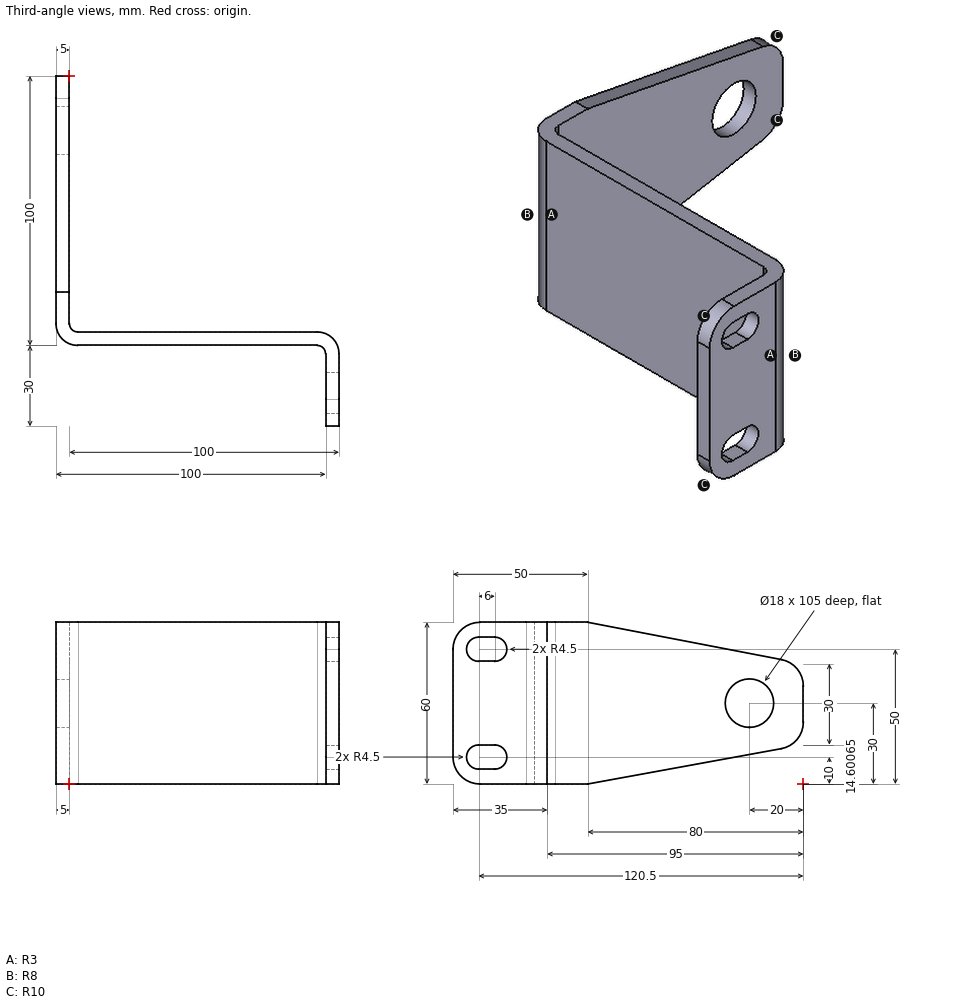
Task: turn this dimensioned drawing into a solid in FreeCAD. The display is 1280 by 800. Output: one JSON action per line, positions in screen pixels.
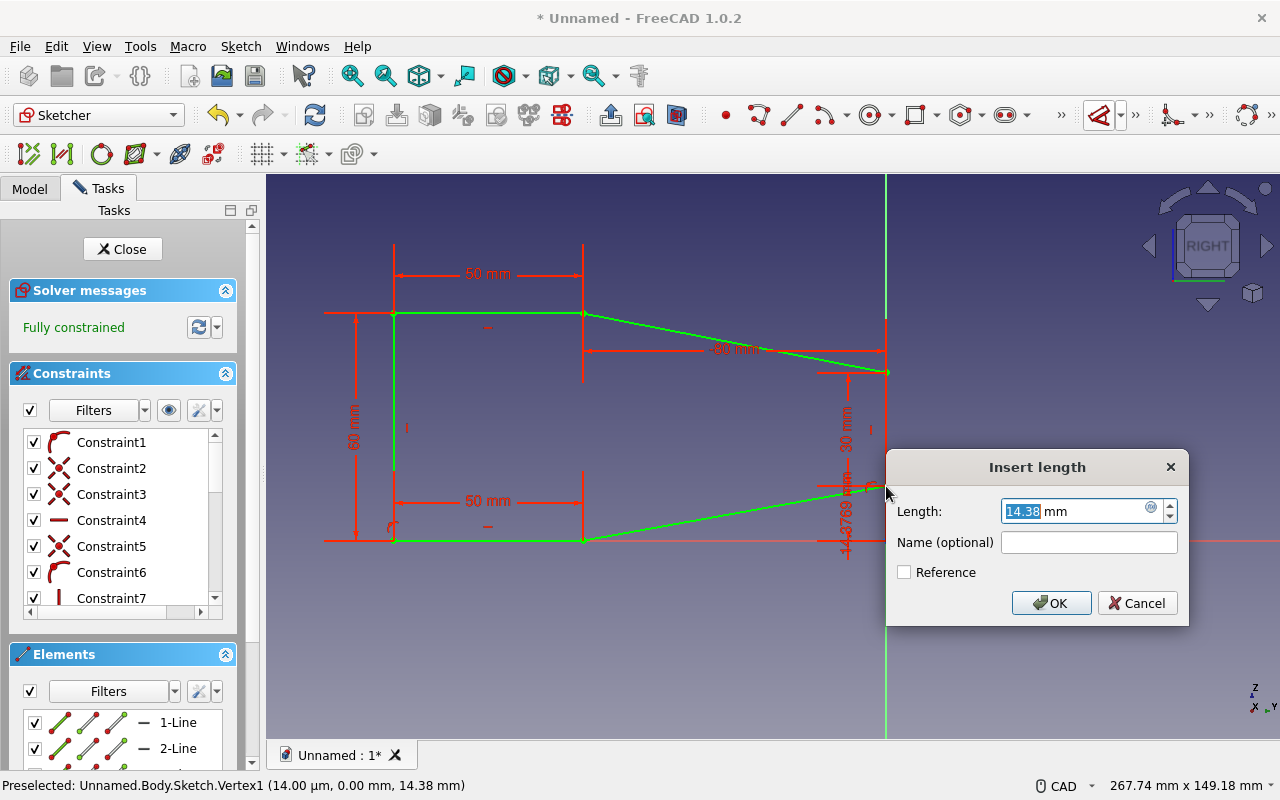
{"action": "type", "text": "14.60065"}
{"action": "key", "text": "Return"}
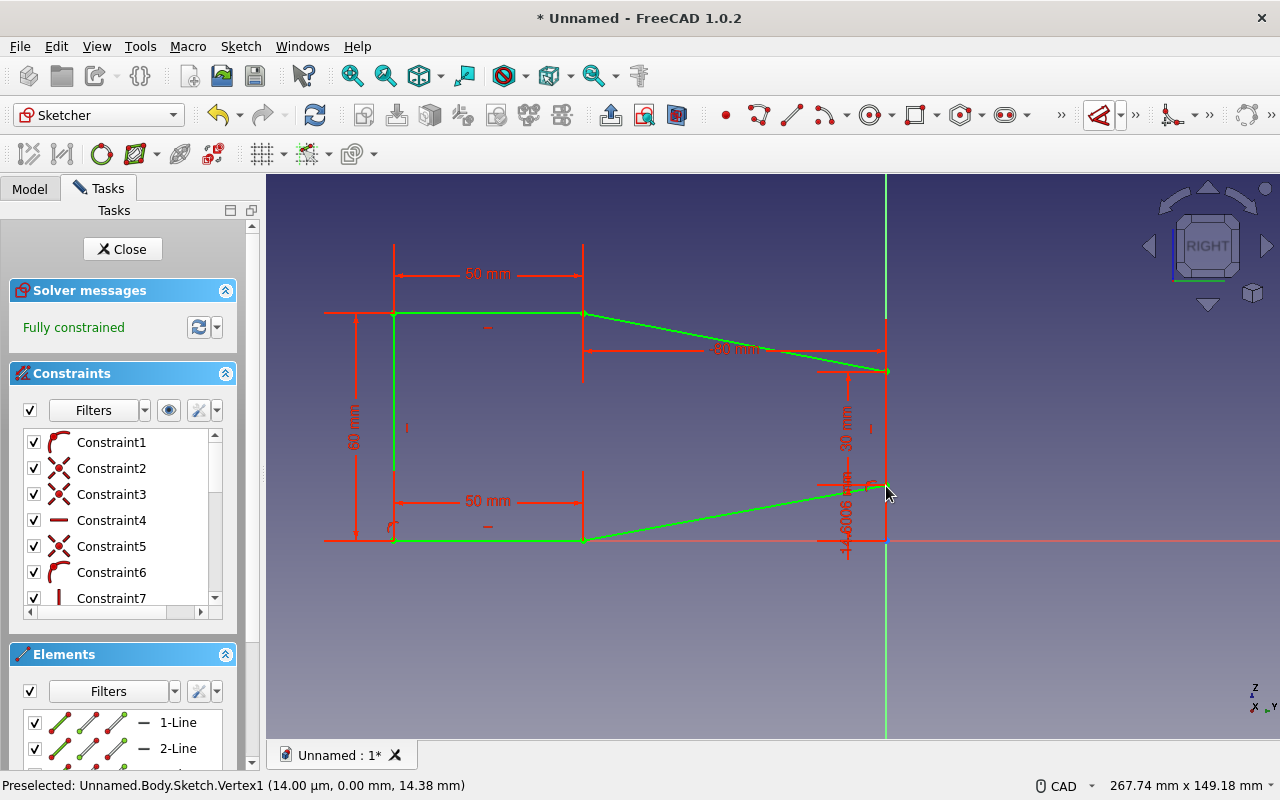
{"action": "left_click", "coordinate": [123, 249]}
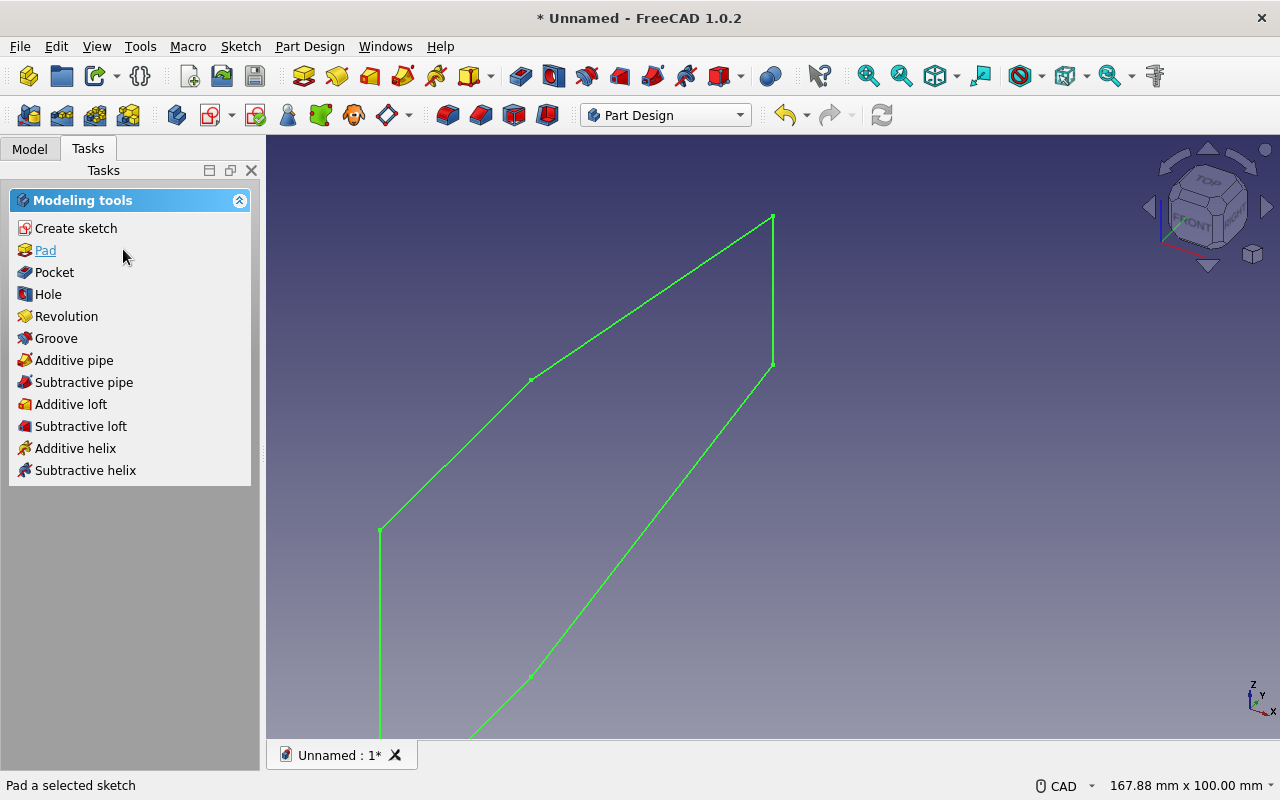
{"action": "left_click", "coordinate": [304, 76]}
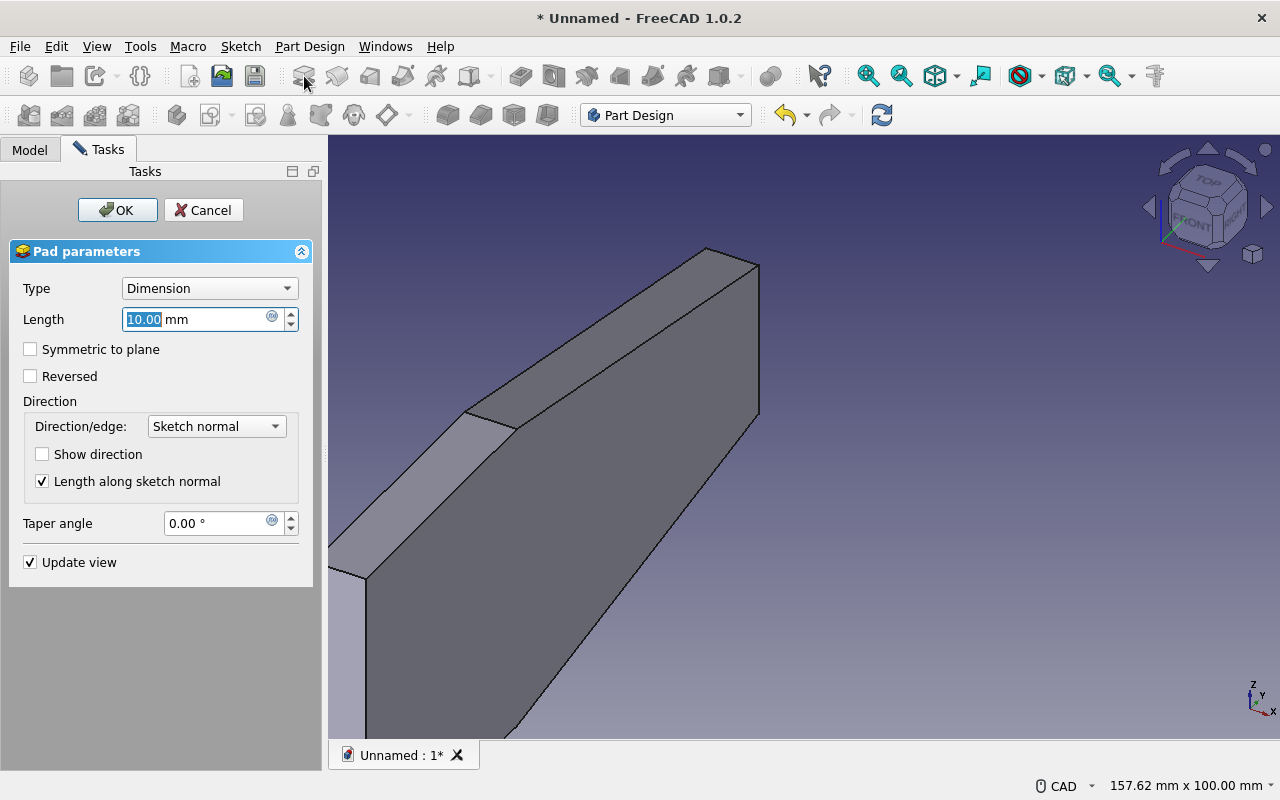
{"action": "type", "text": "5"}
{"action": "key", "text": "Tab"}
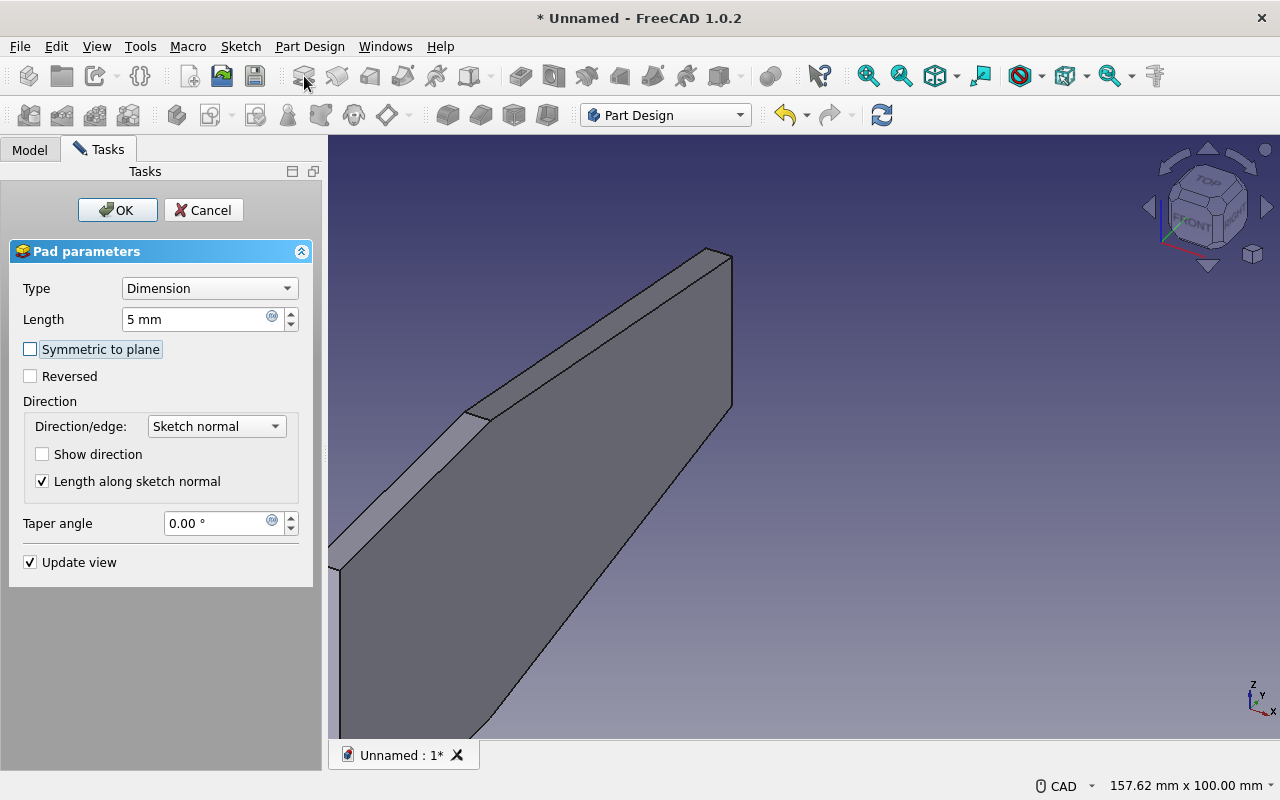
{"action": "left_click", "coordinate": [31, 376]}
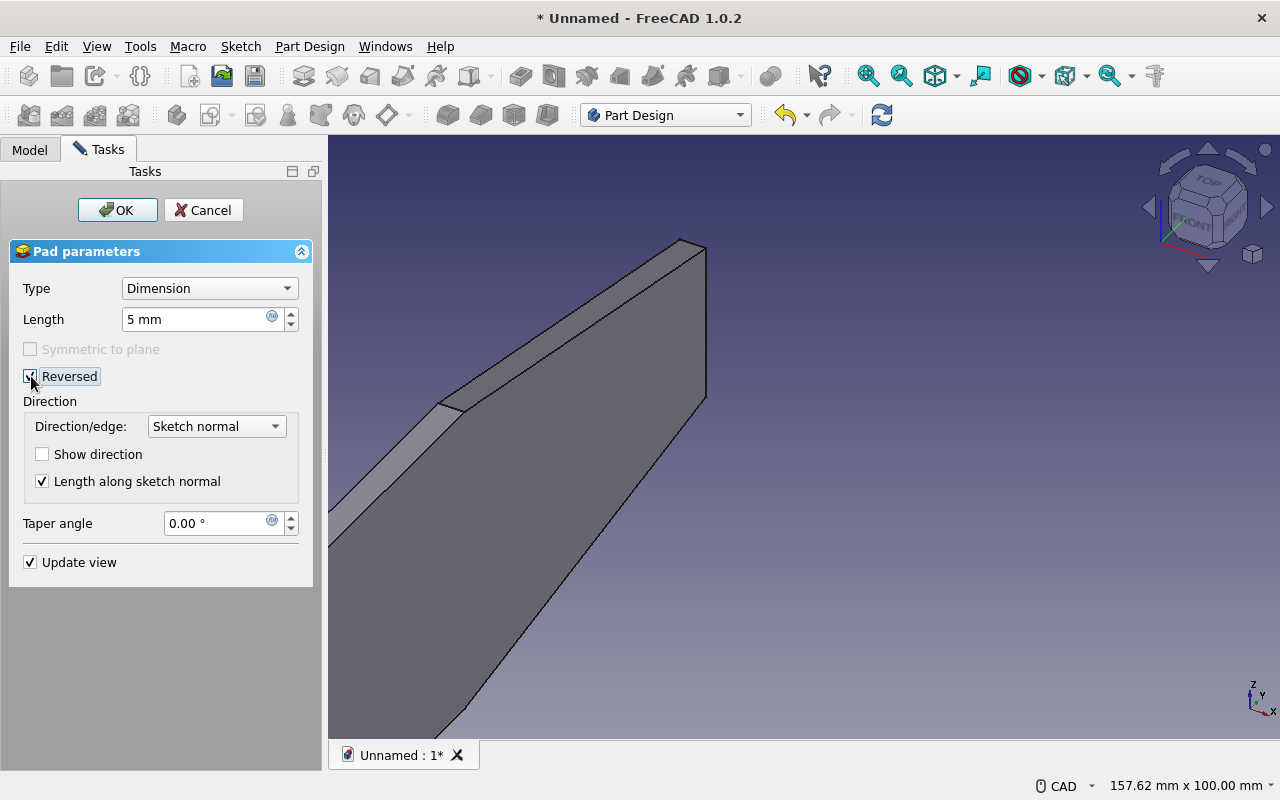
{"action": "left_click", "coordinate": [118, 210]}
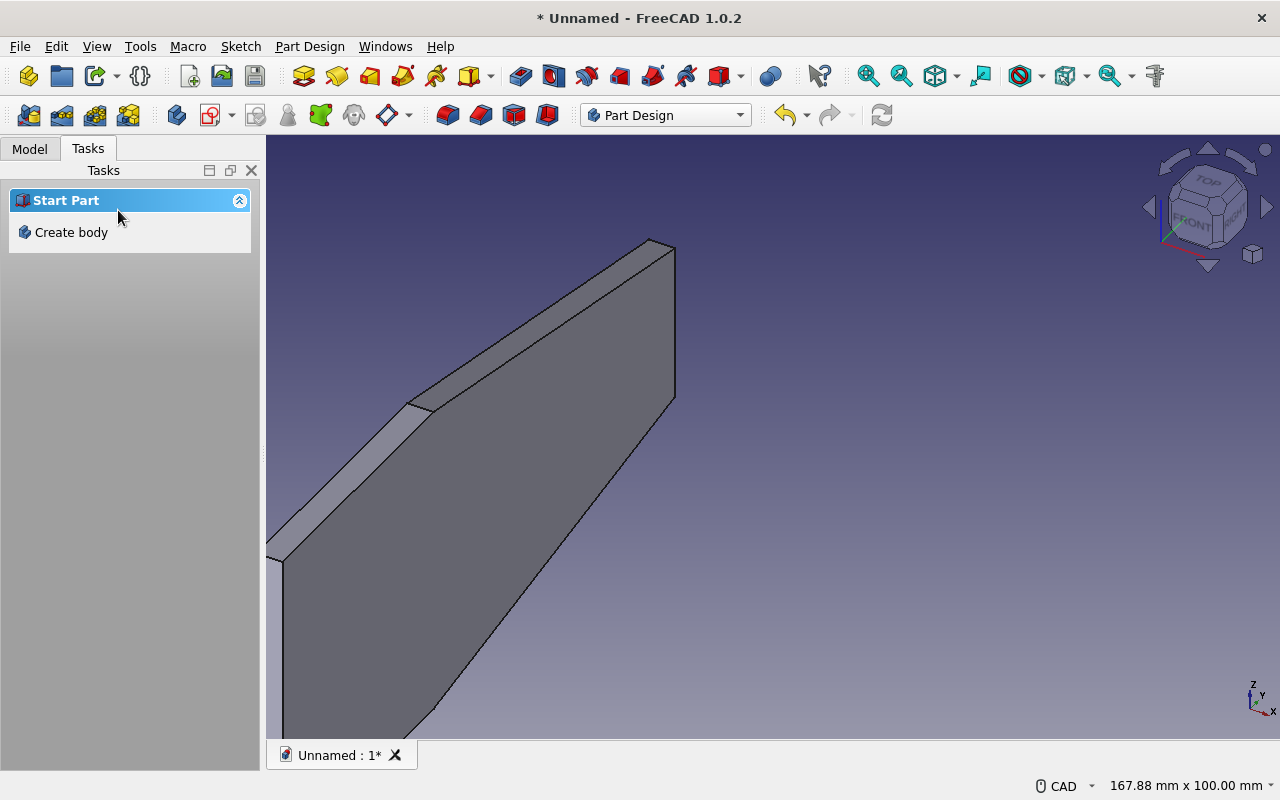
{"action": "left_click", "coordinate": [869, 76]}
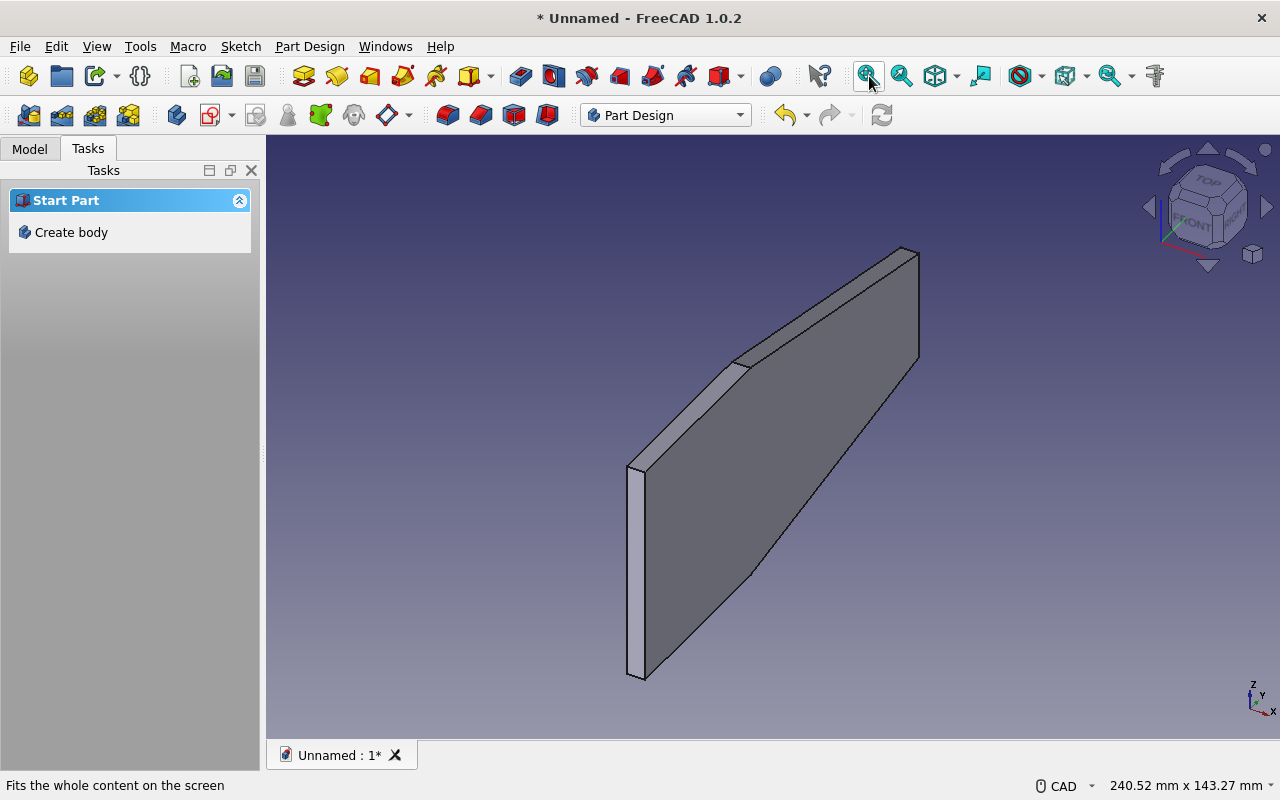
{"action": "left_click", "coordinate": [210, 116]}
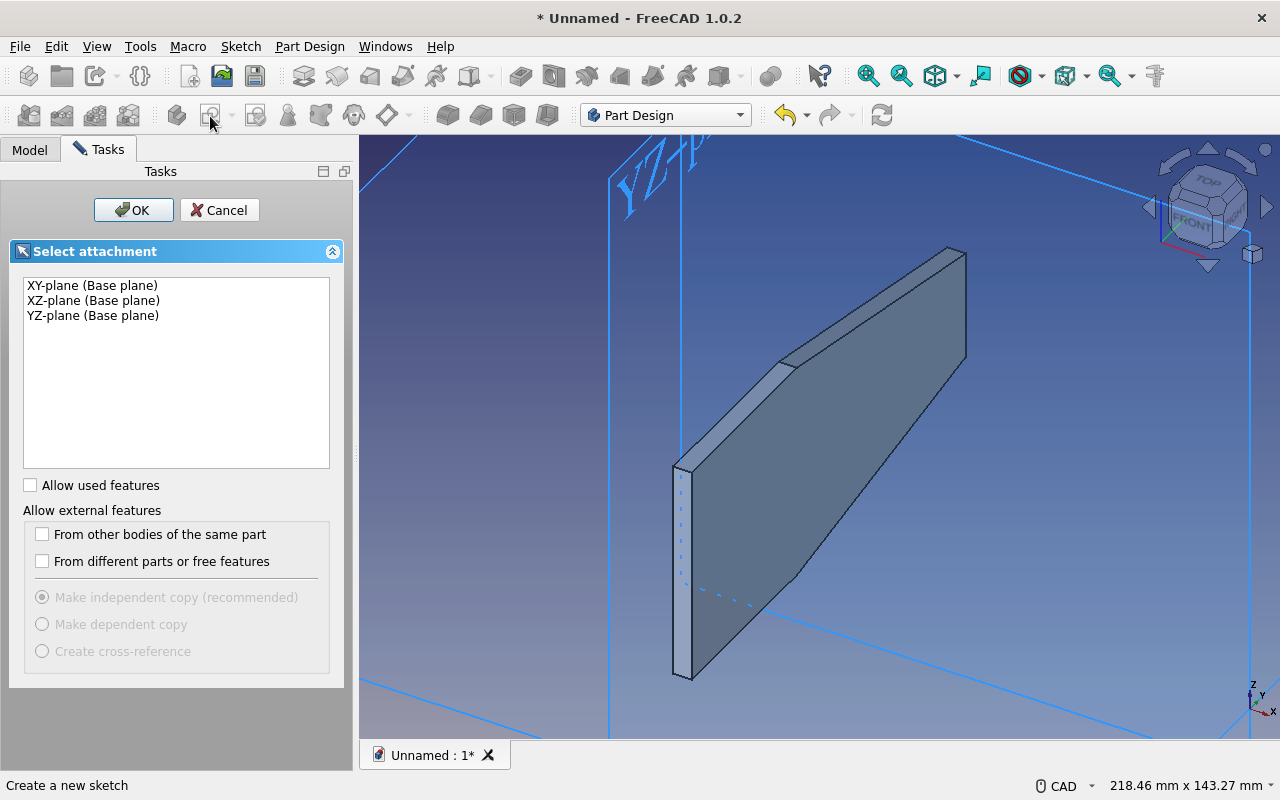
{"action": "left_click", "coordinate": [84, 316]}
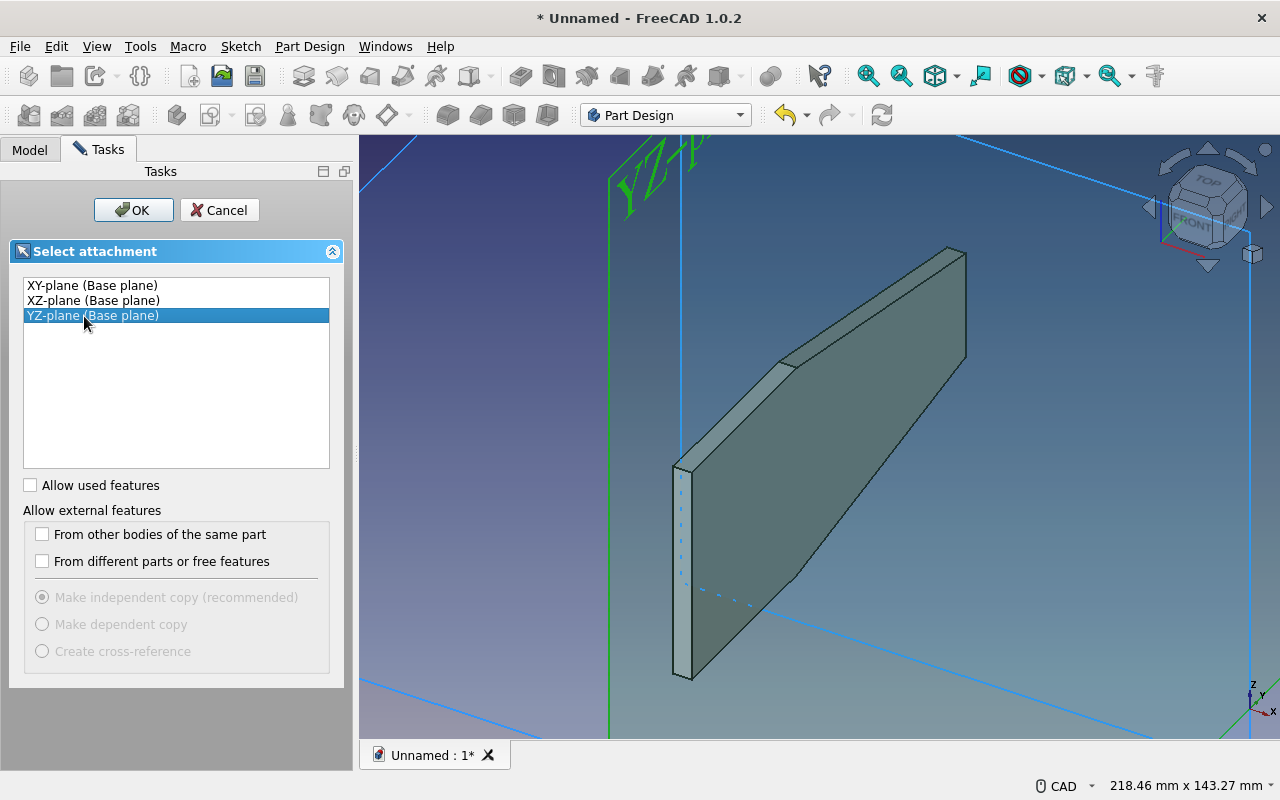
{"action": "left_click", "coordinate": [134, 210]}